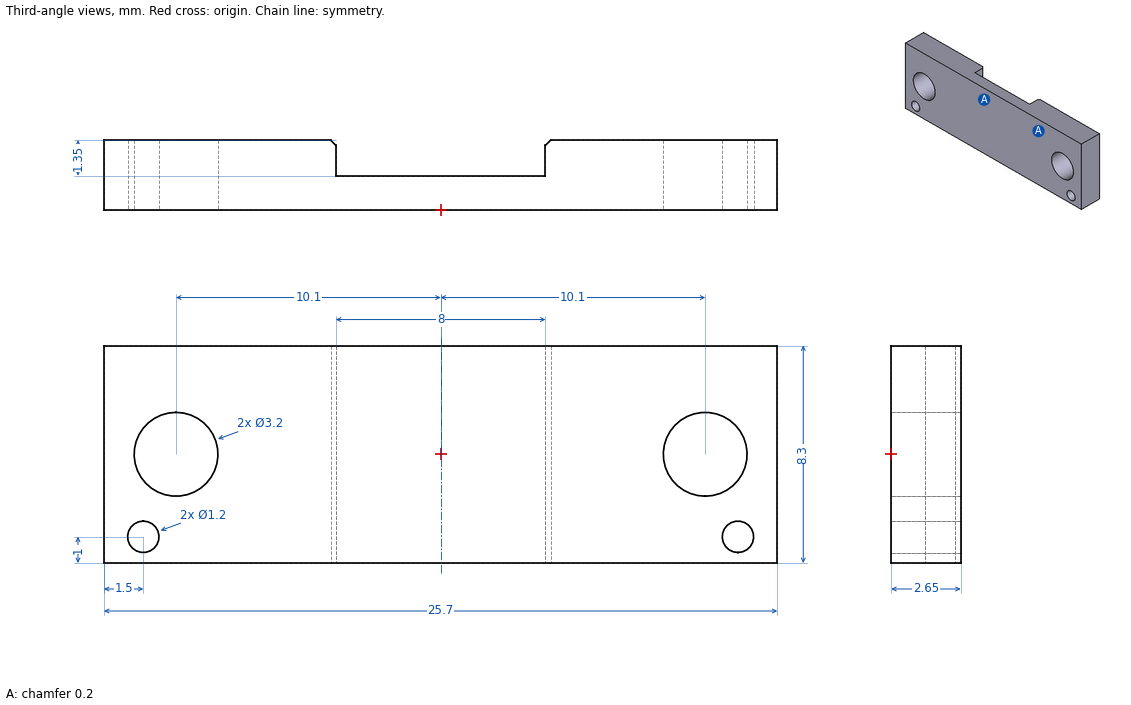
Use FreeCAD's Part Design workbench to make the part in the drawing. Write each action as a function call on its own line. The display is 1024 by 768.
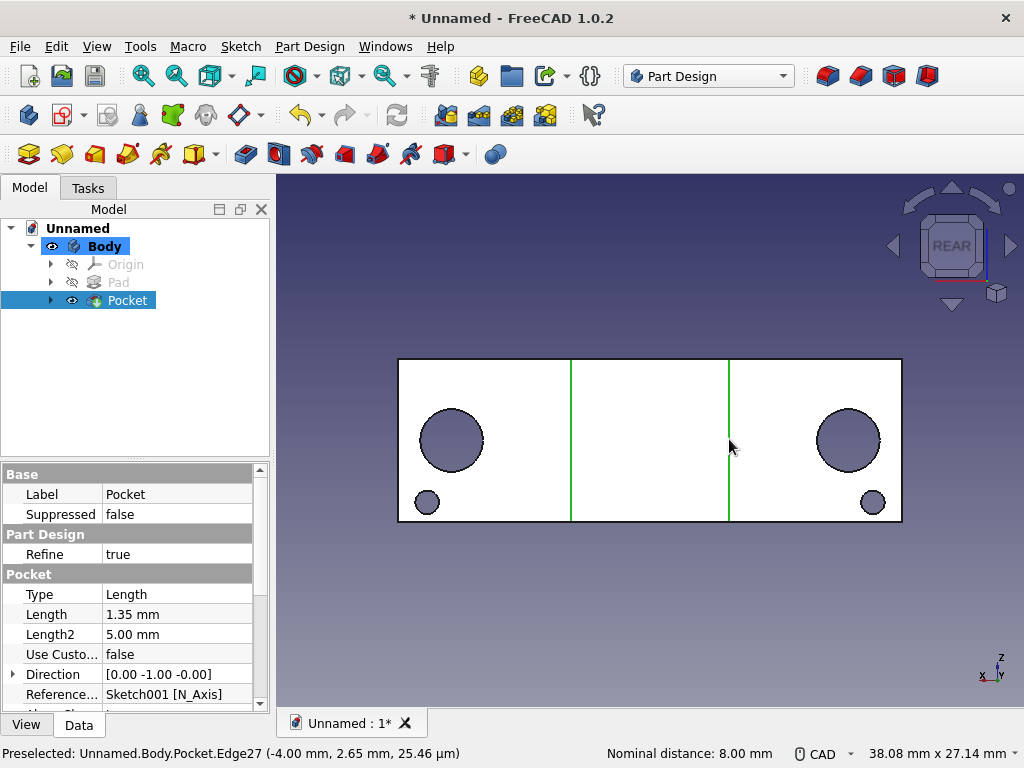
click(861, 76)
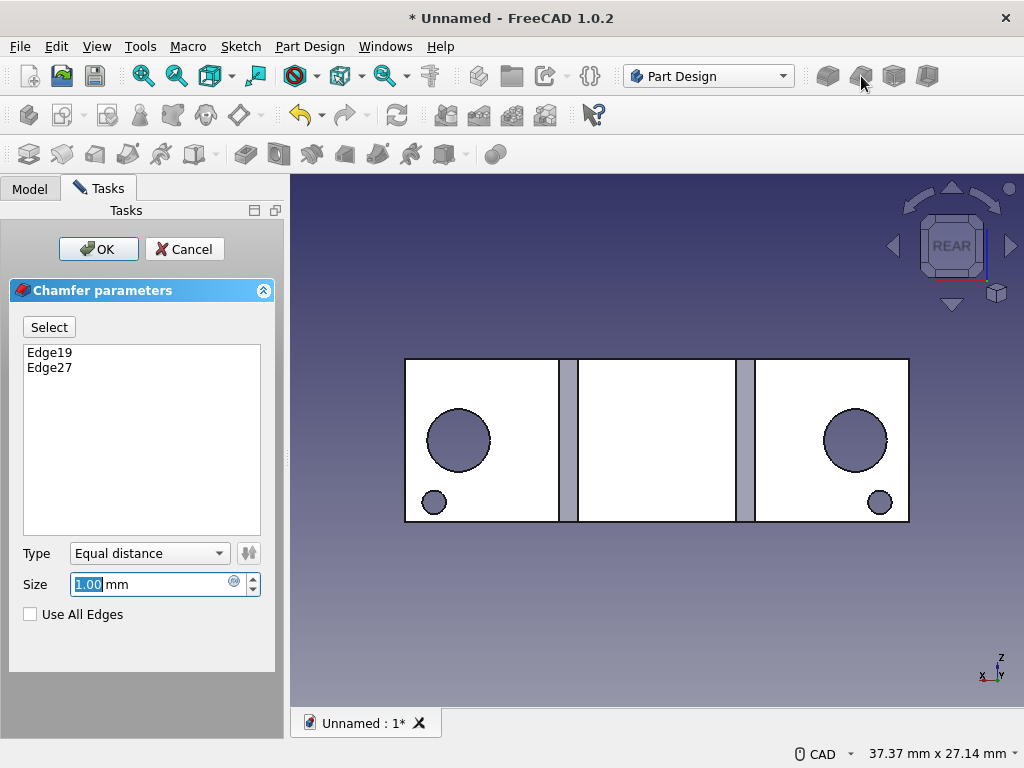
text(0.2)
key(Tab)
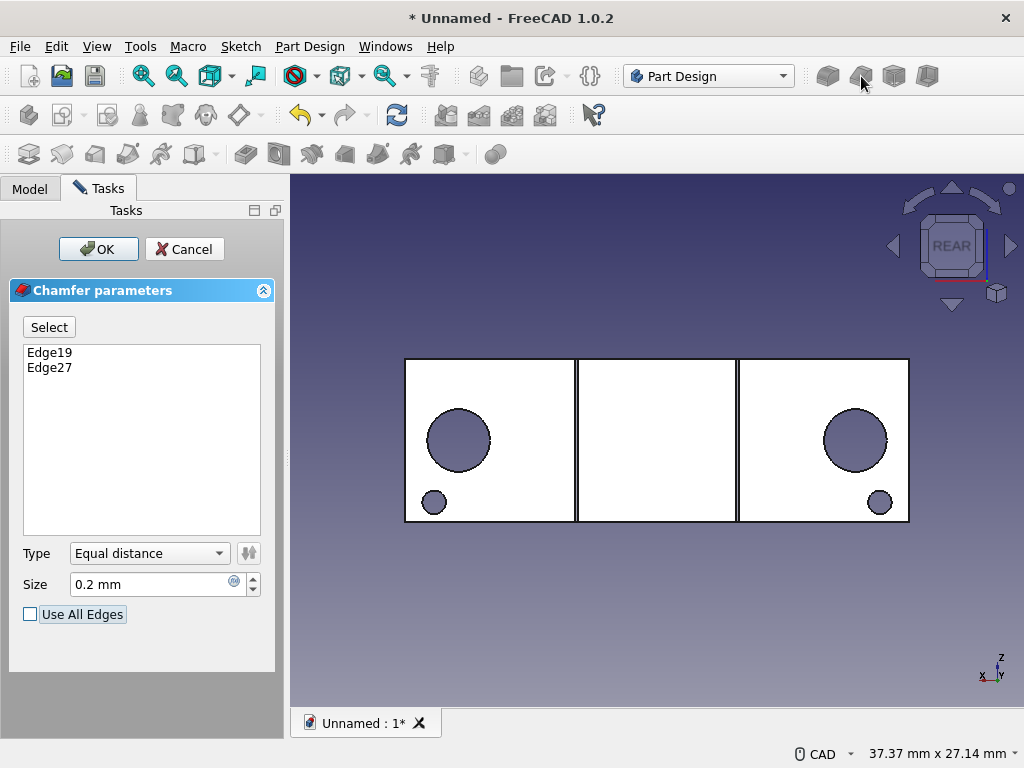
click(99, 249)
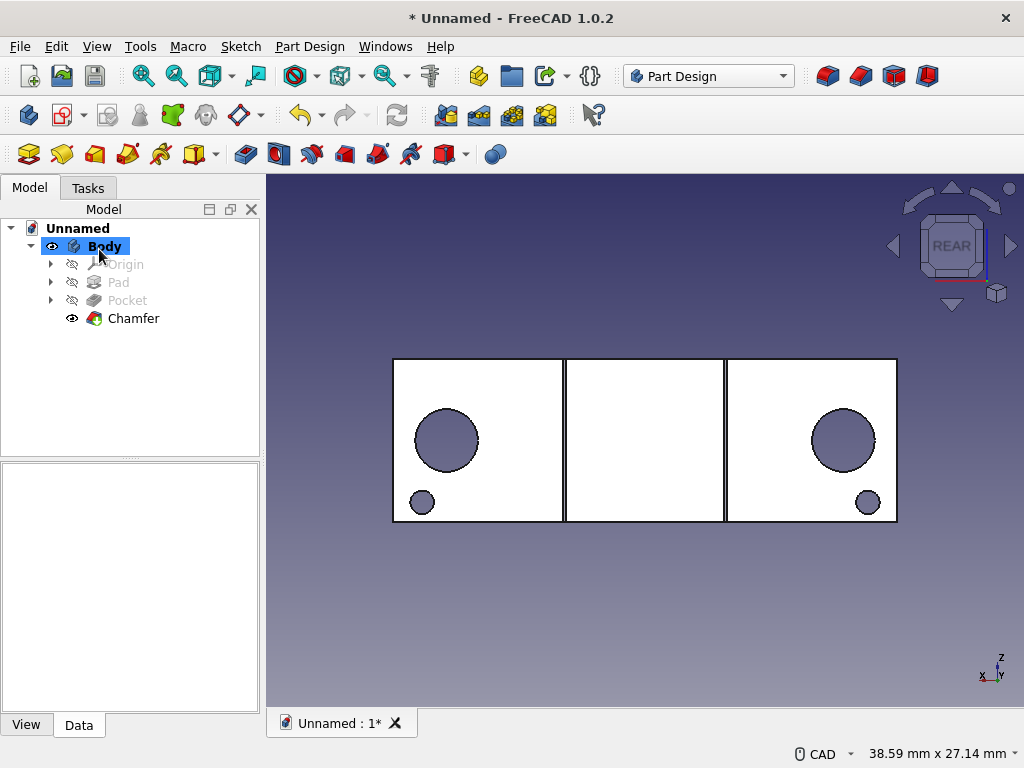
key(0)